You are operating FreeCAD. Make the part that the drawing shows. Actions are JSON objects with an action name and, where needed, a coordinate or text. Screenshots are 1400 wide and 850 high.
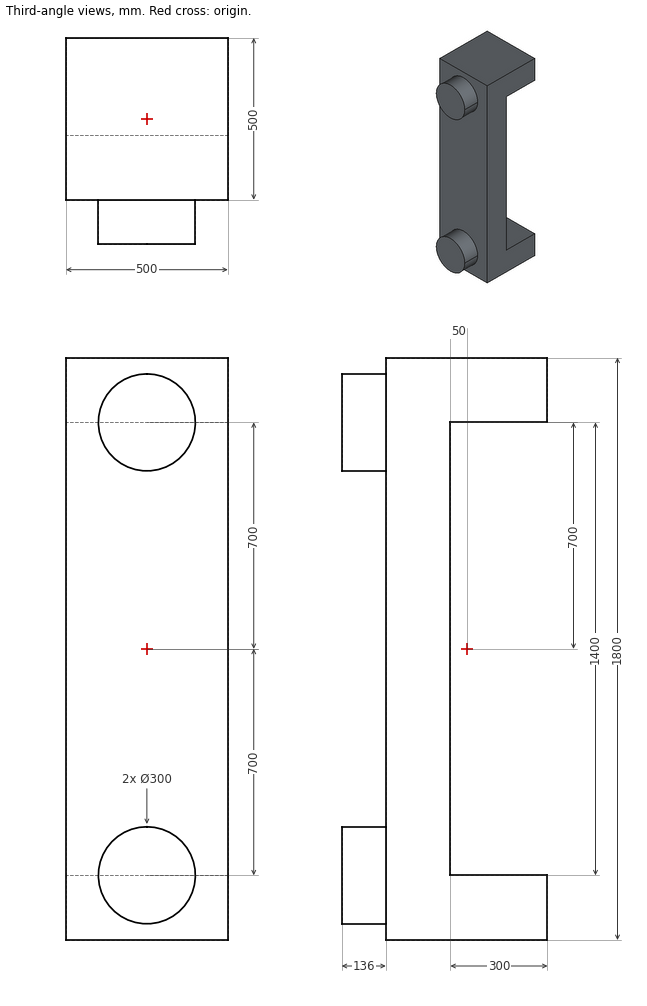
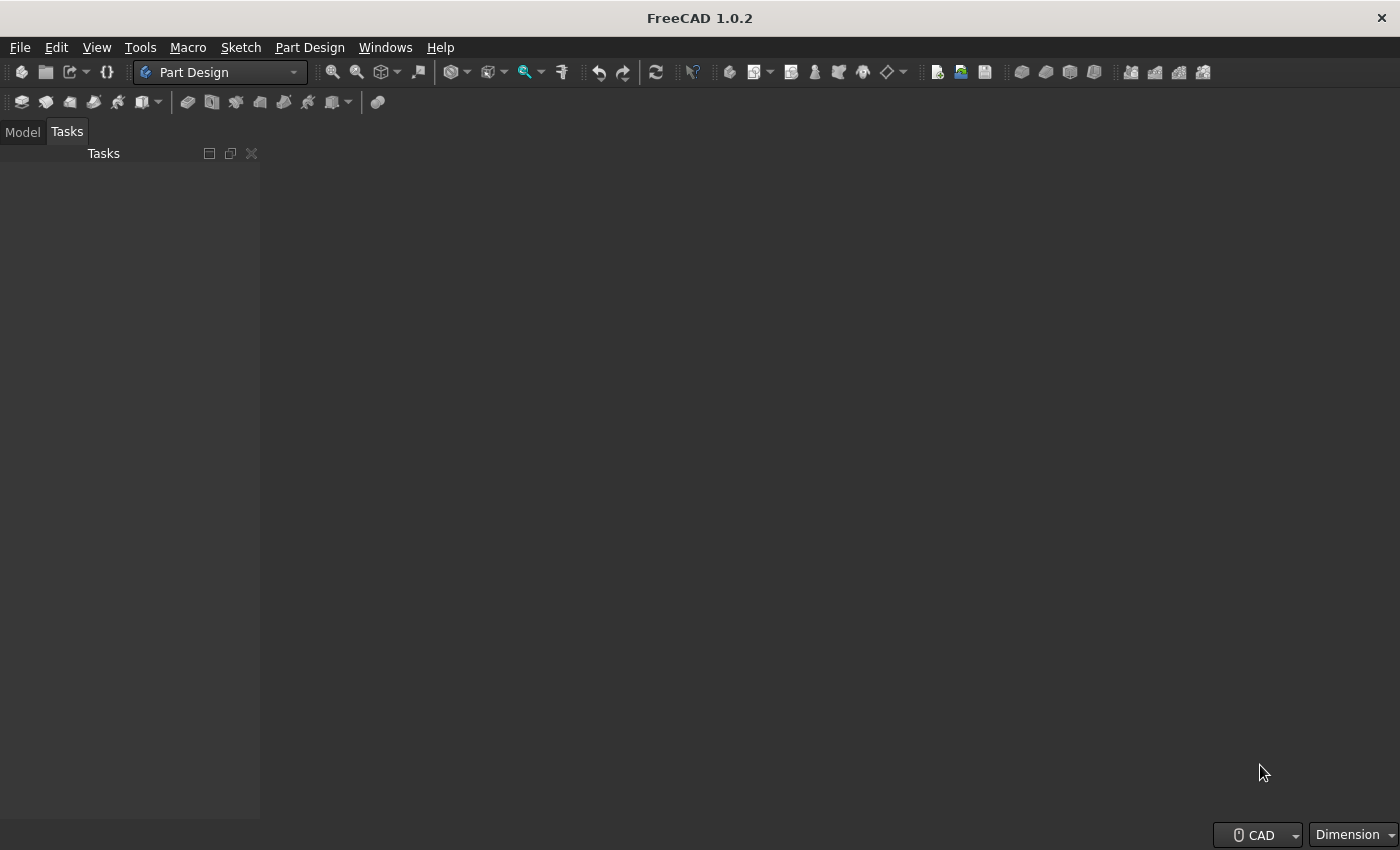
{"action": "left_click", "coordinate": [938, 72]}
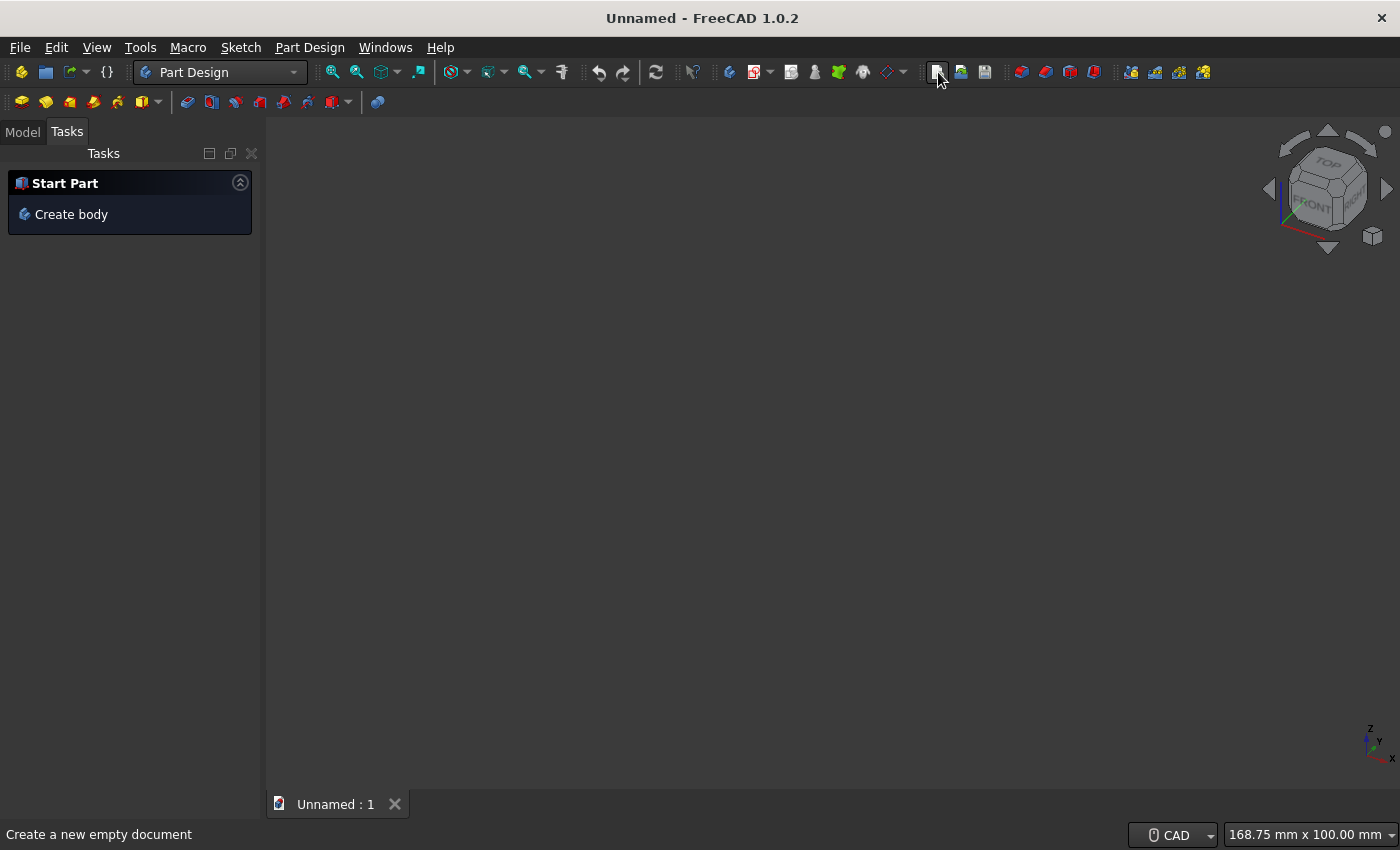
{"action": "left_click", "coordinate": [754, 72]}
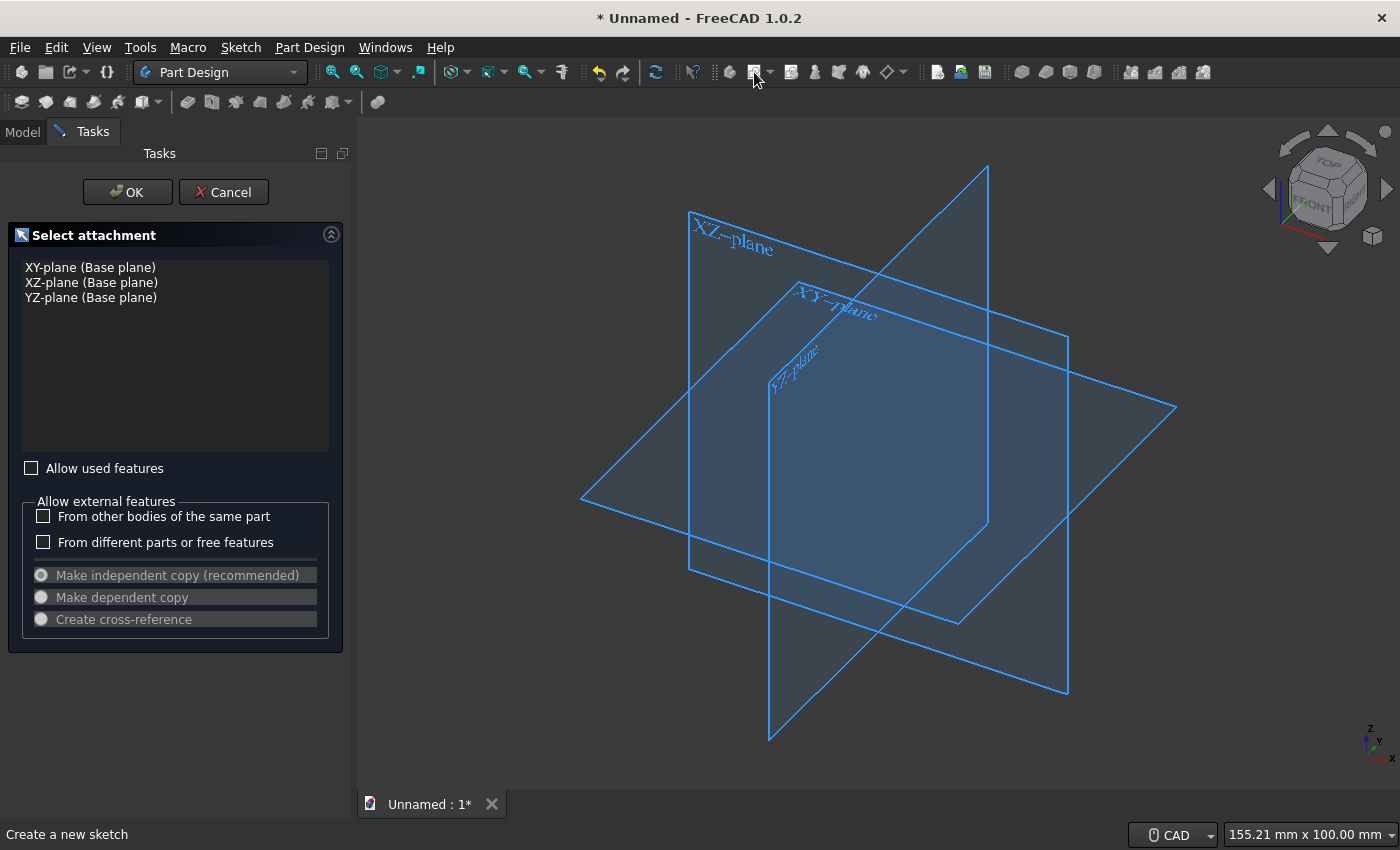
{"action": "left_click", "coordinate": [82, 268]}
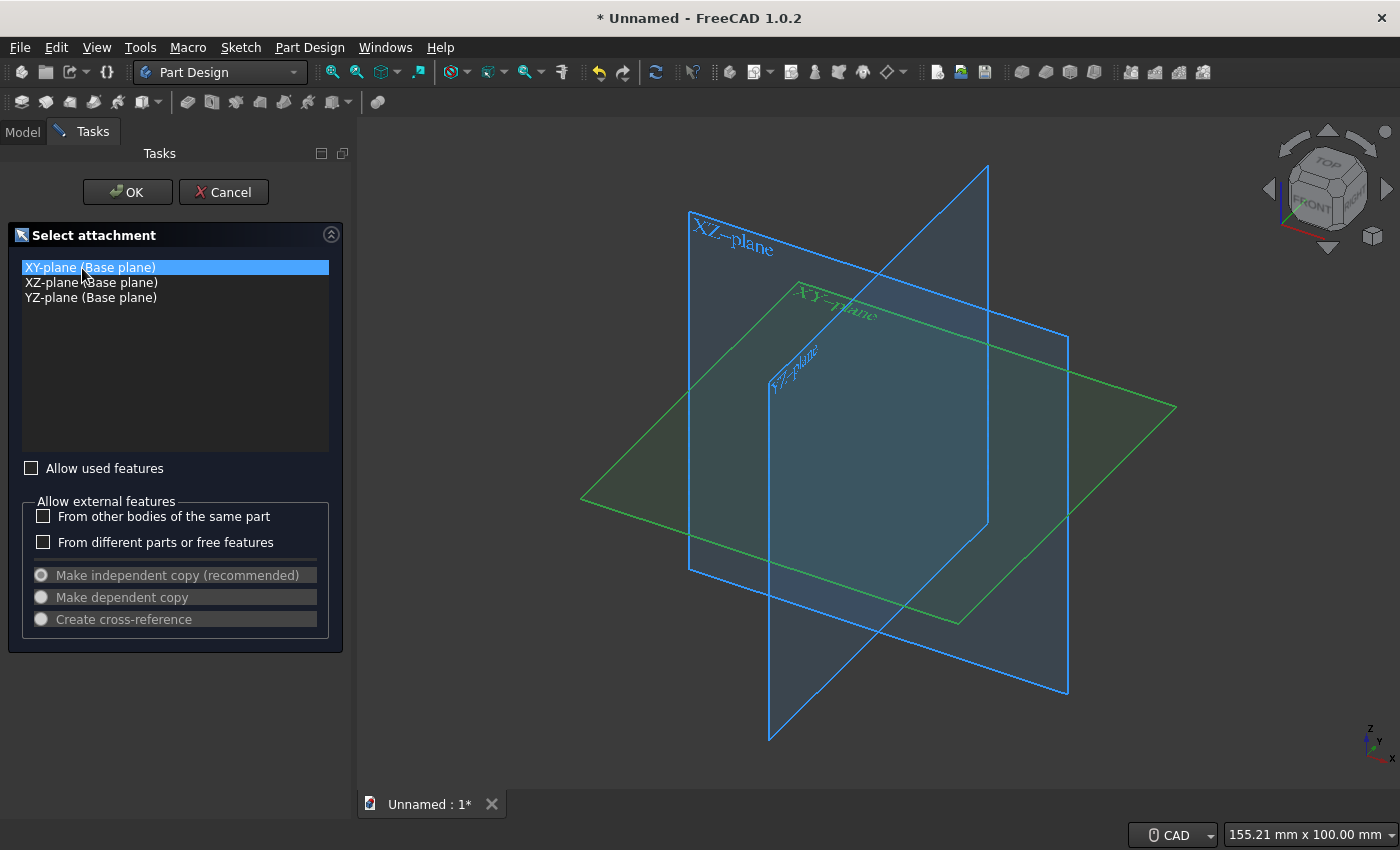
{"action": "left_click", "coordinate": [128, 192]}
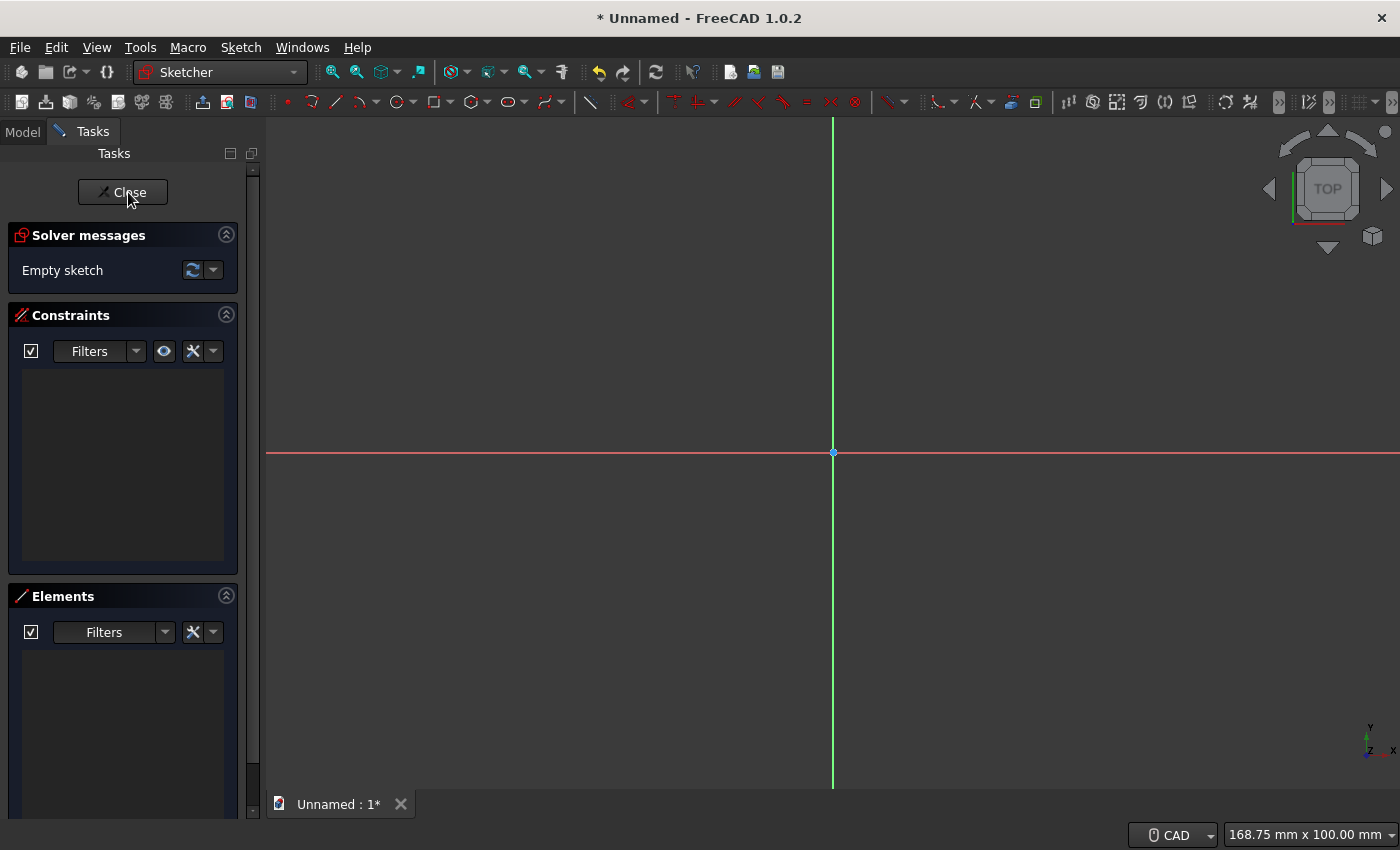
{"action": "scroll", "coordinate": [754, 453], "scroll_direction": "down", "scroll_amount": 10}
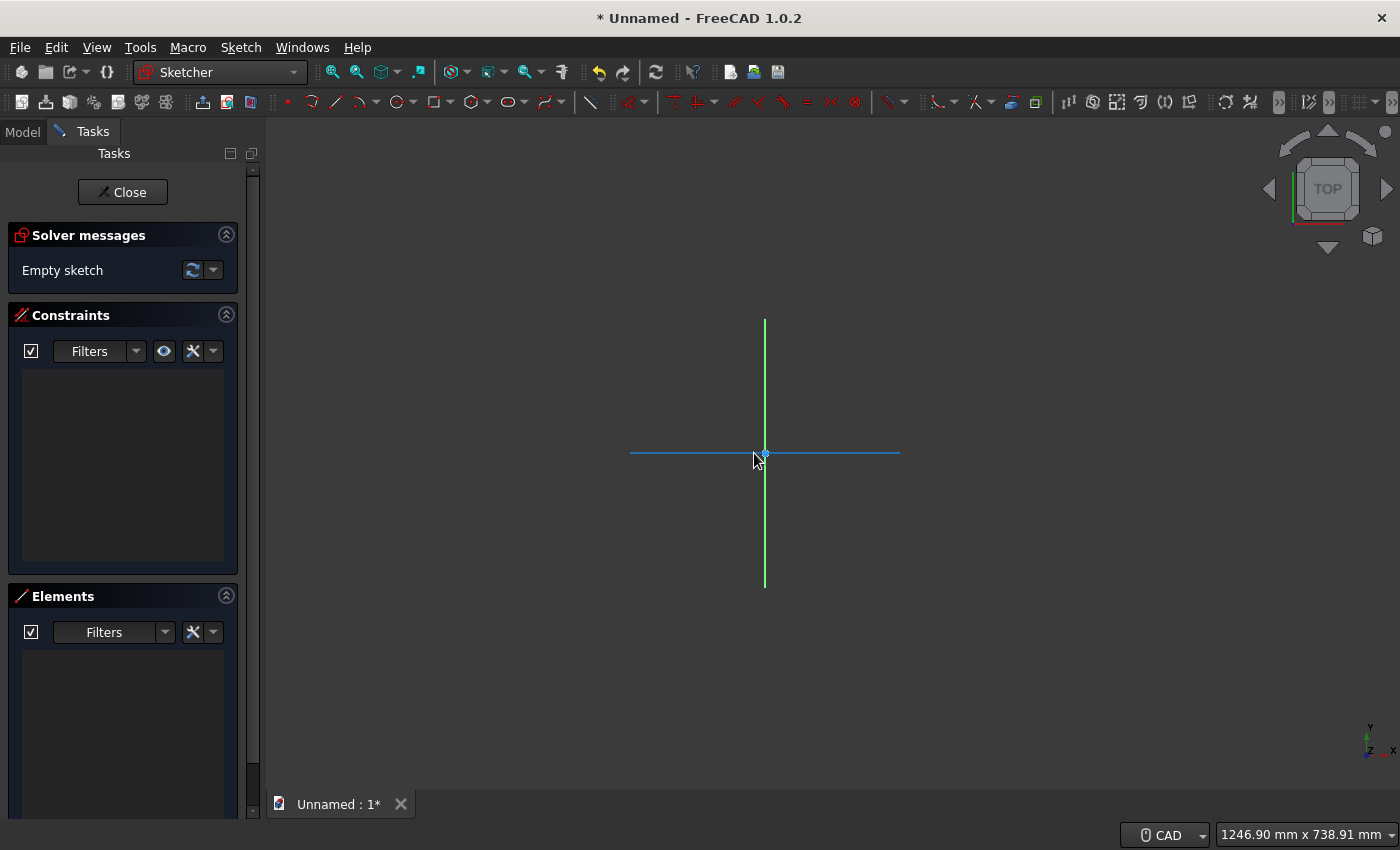
{"action": "key", "text": "g v"}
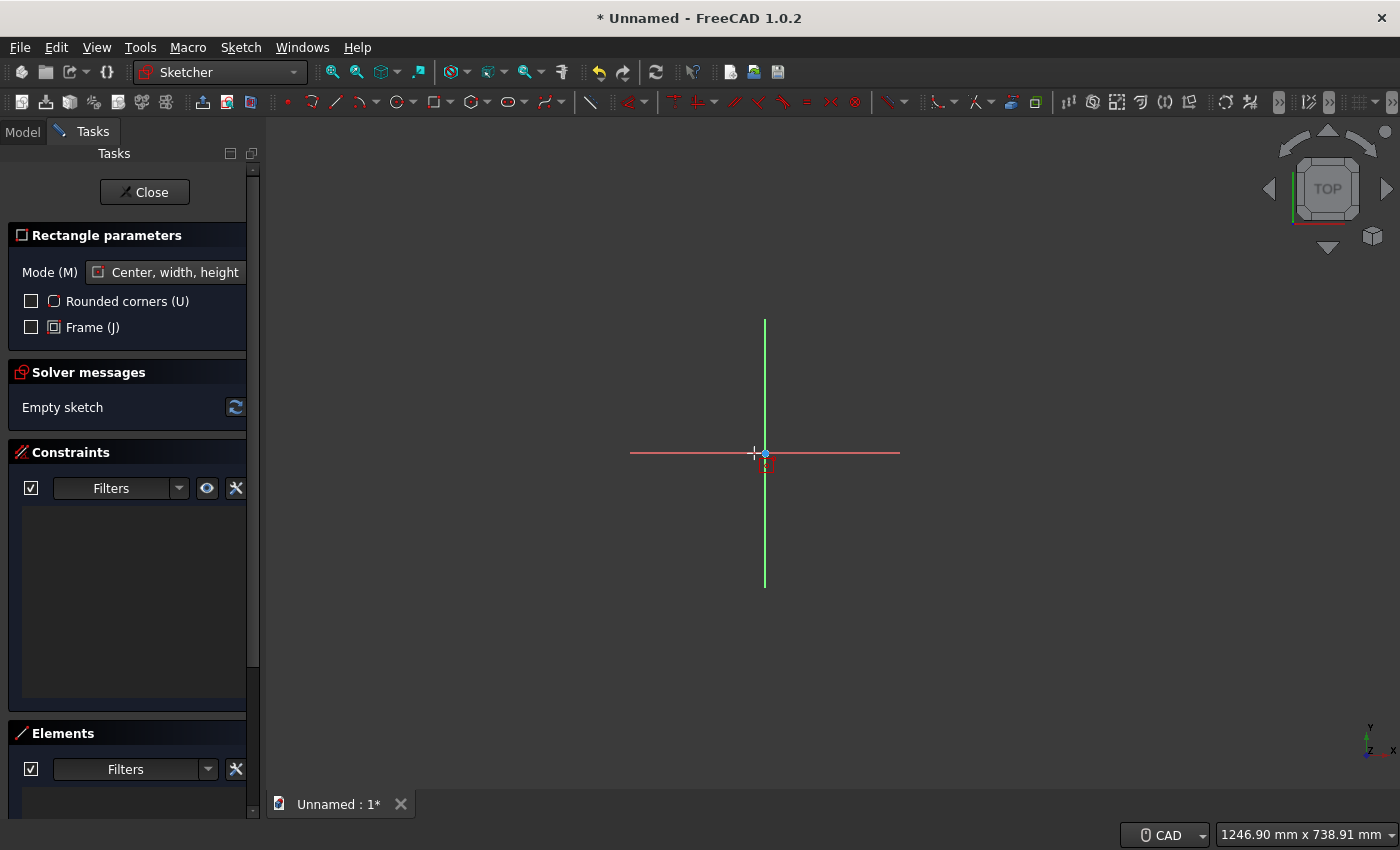
{"action": "left_click", "coordinate": [765, 453]}
{"action": "left_click", "coordinate": [992, 226]}
{"action": "key", "text": "Escape"}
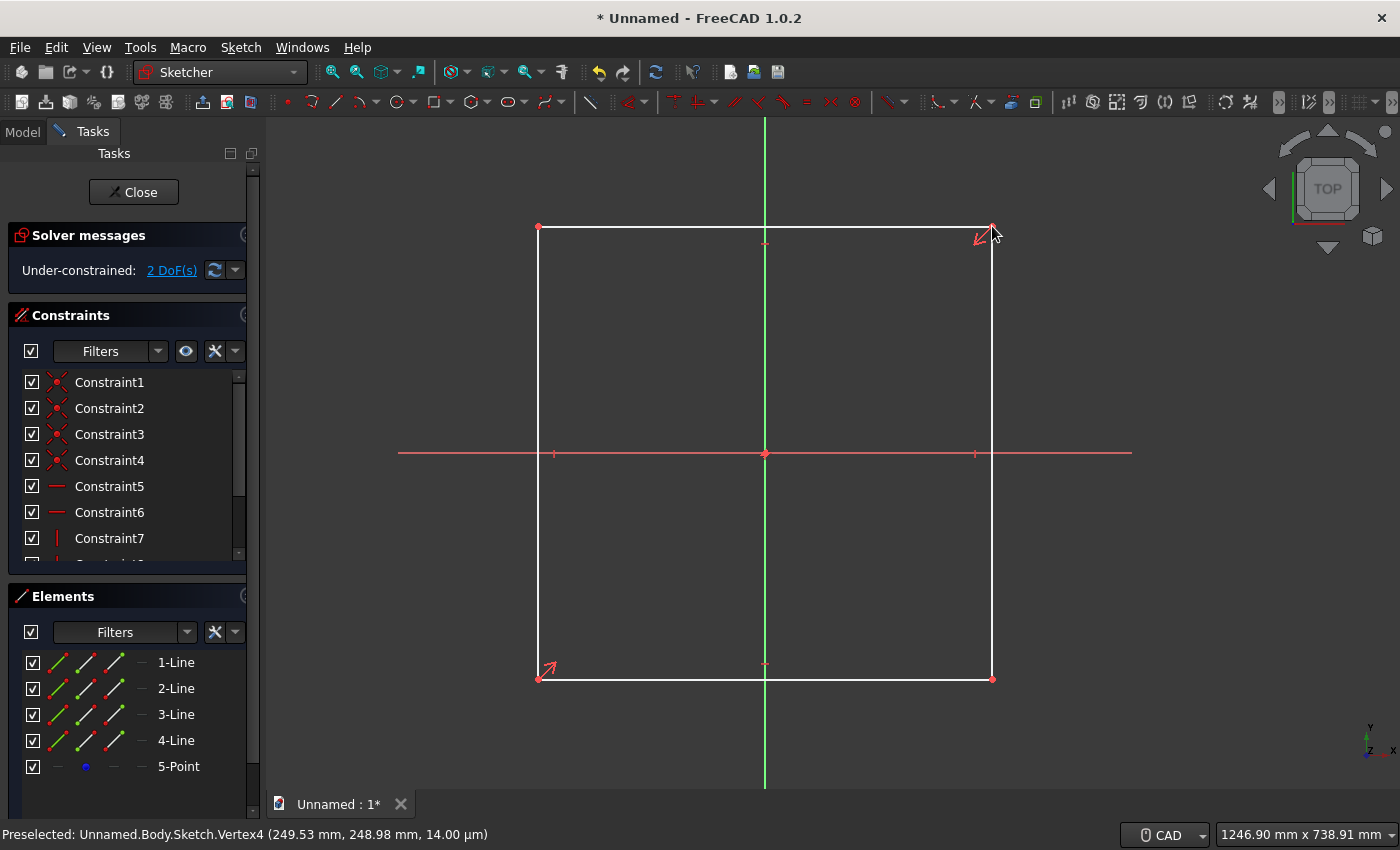
{"action": "left_click", "coordinate": [628, 102]}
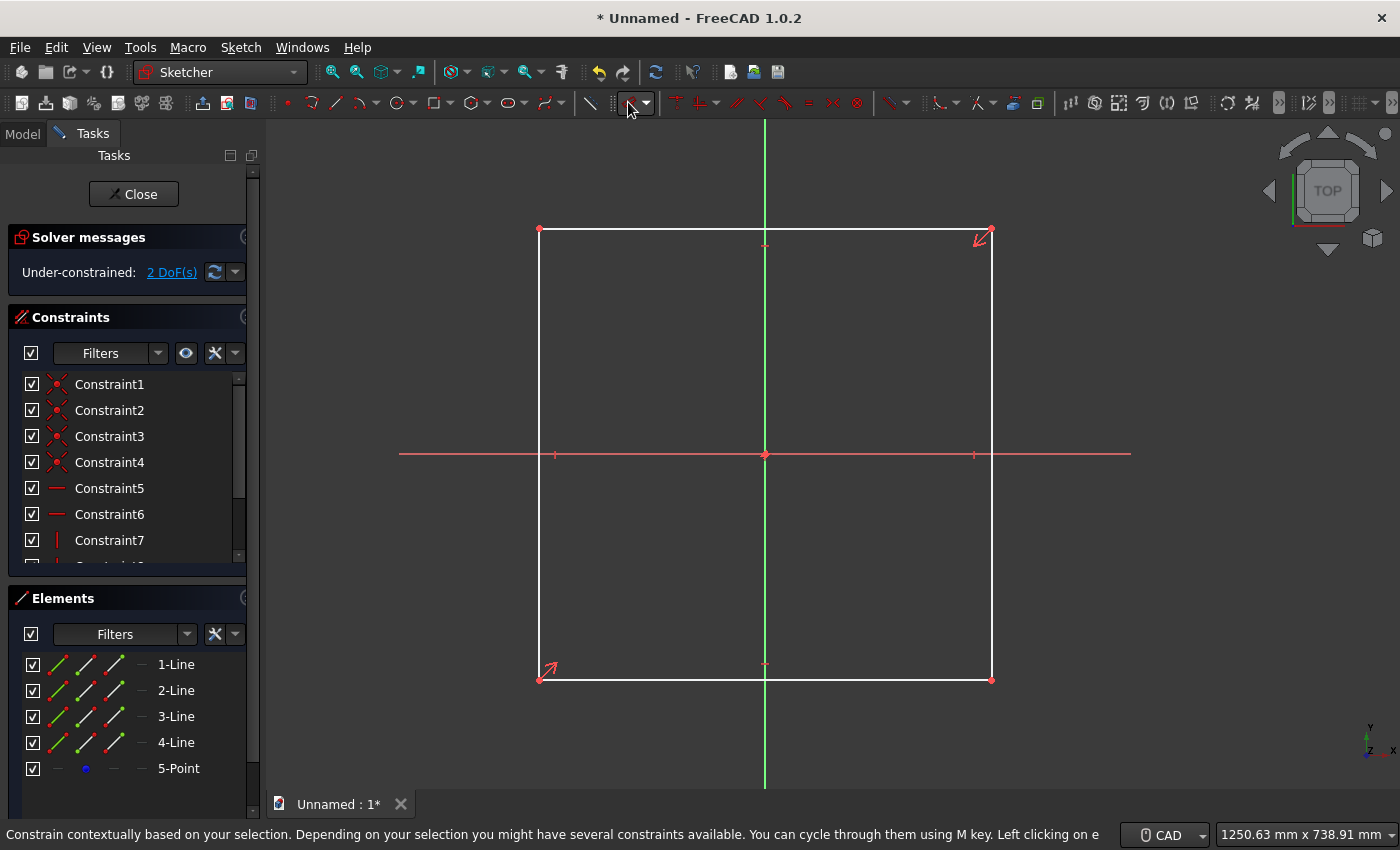
{"action": "left_click", "coordinate": [675, 680]}
{"action": "left_click", "coordinate": [661, 714]}